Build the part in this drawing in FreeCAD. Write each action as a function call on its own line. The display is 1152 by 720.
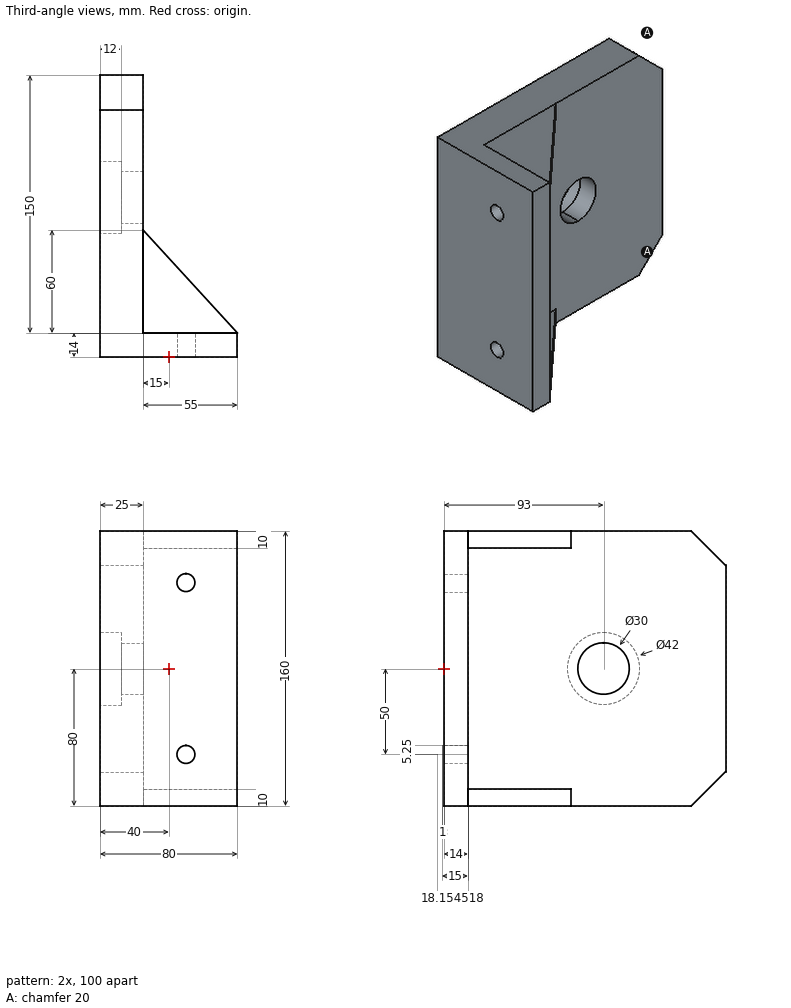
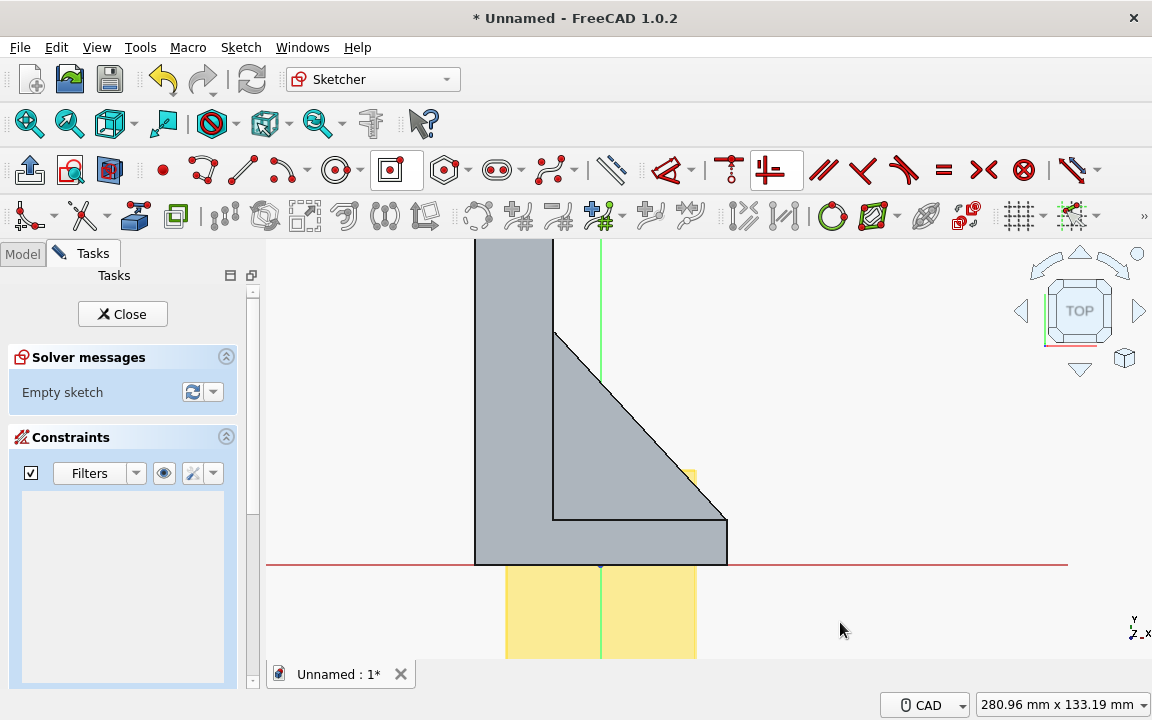
click(204, 170)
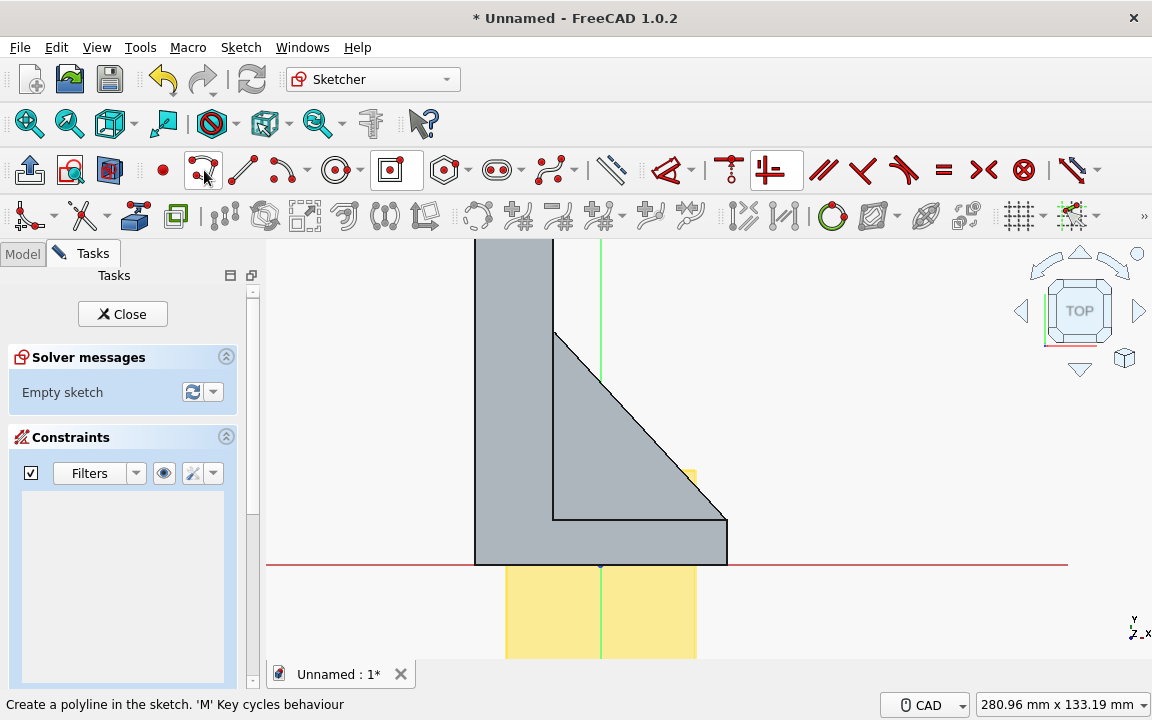
click(553, 520)
click(553, 331)
click(727, 520)
click(553, 521)
key(Escape)
key(Escape)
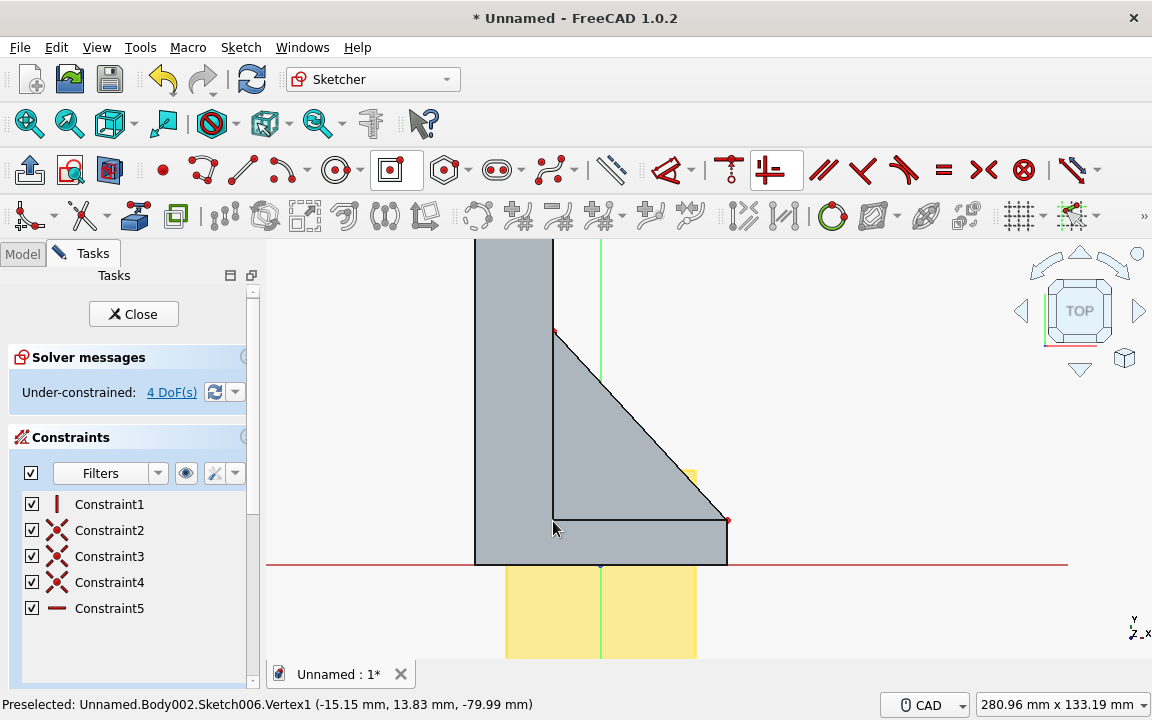
key(d)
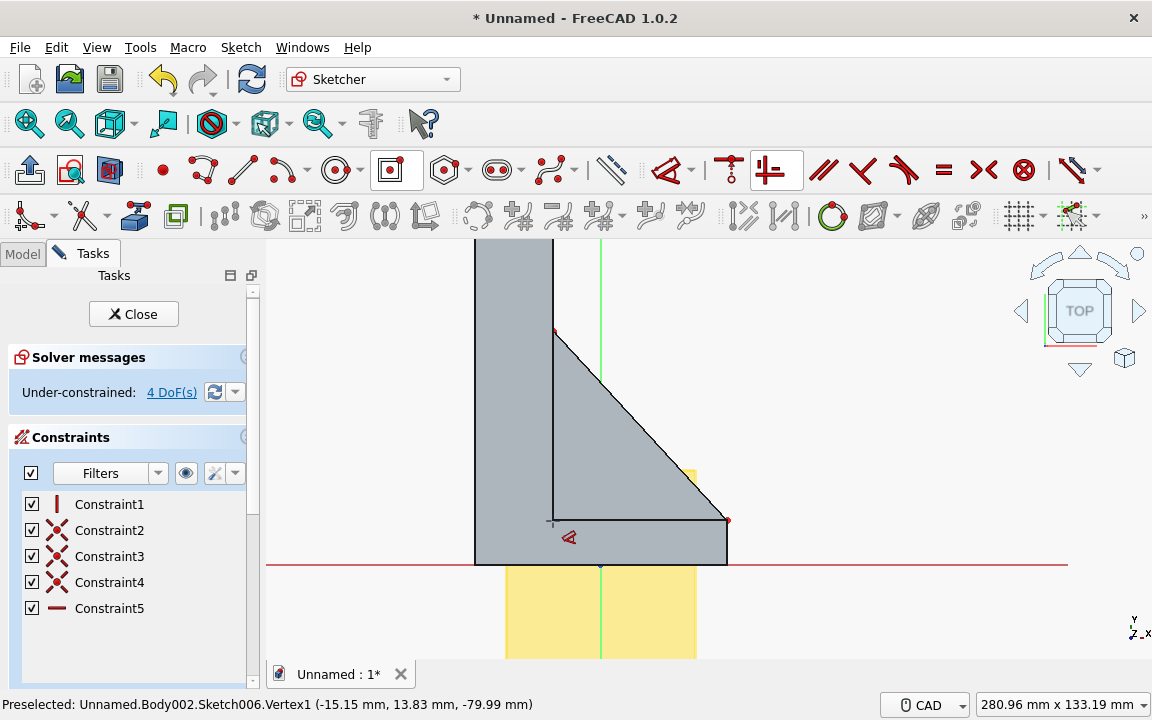
click(553, 464)
click(519, 427)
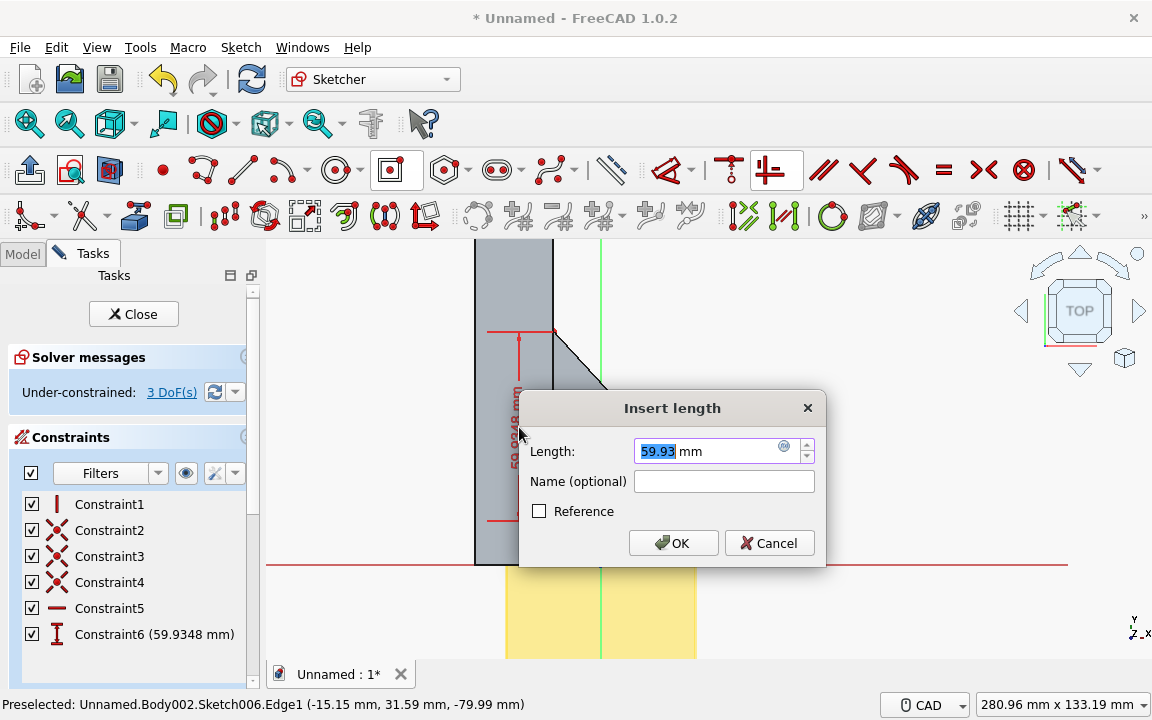
text(60)
key(Return)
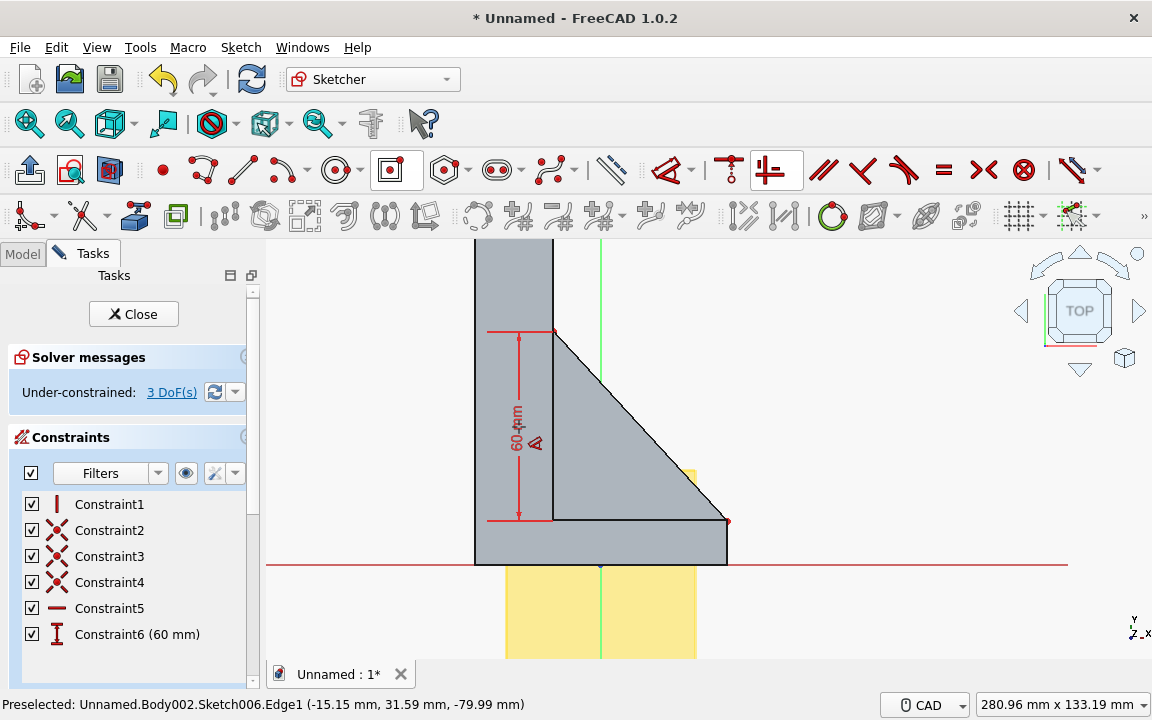
click(675, 521)
click(640, 487)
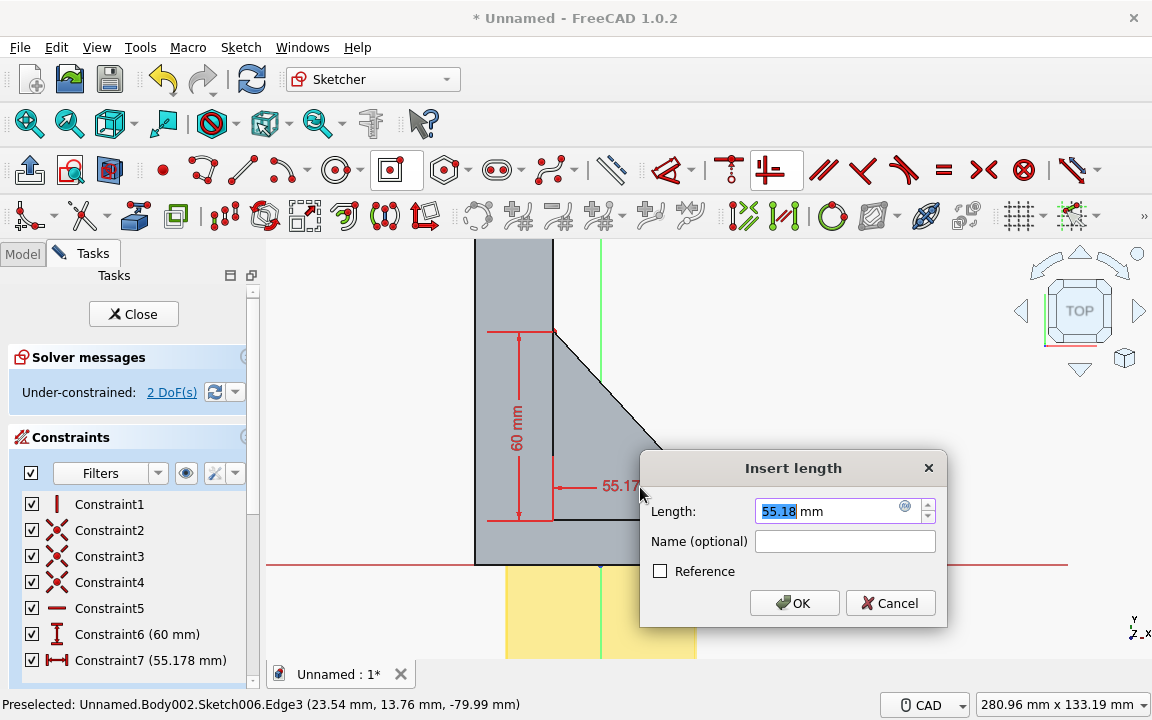
text(55)
key(Return)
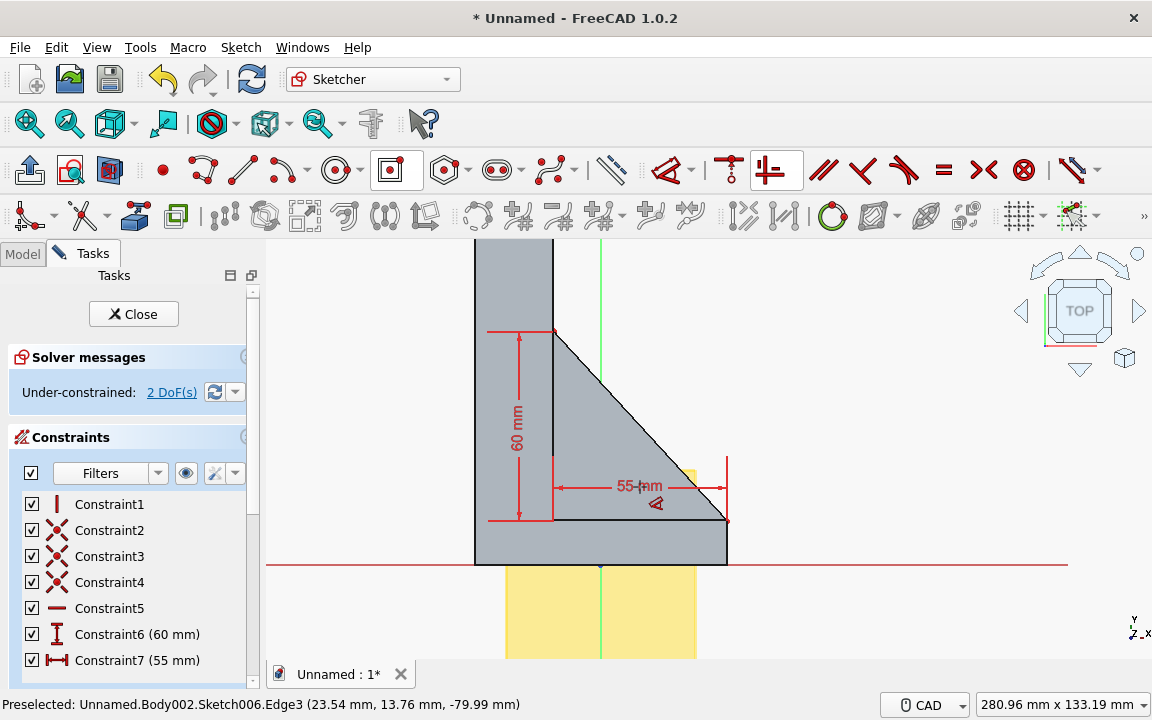
click(553, 521)
click(577, 599)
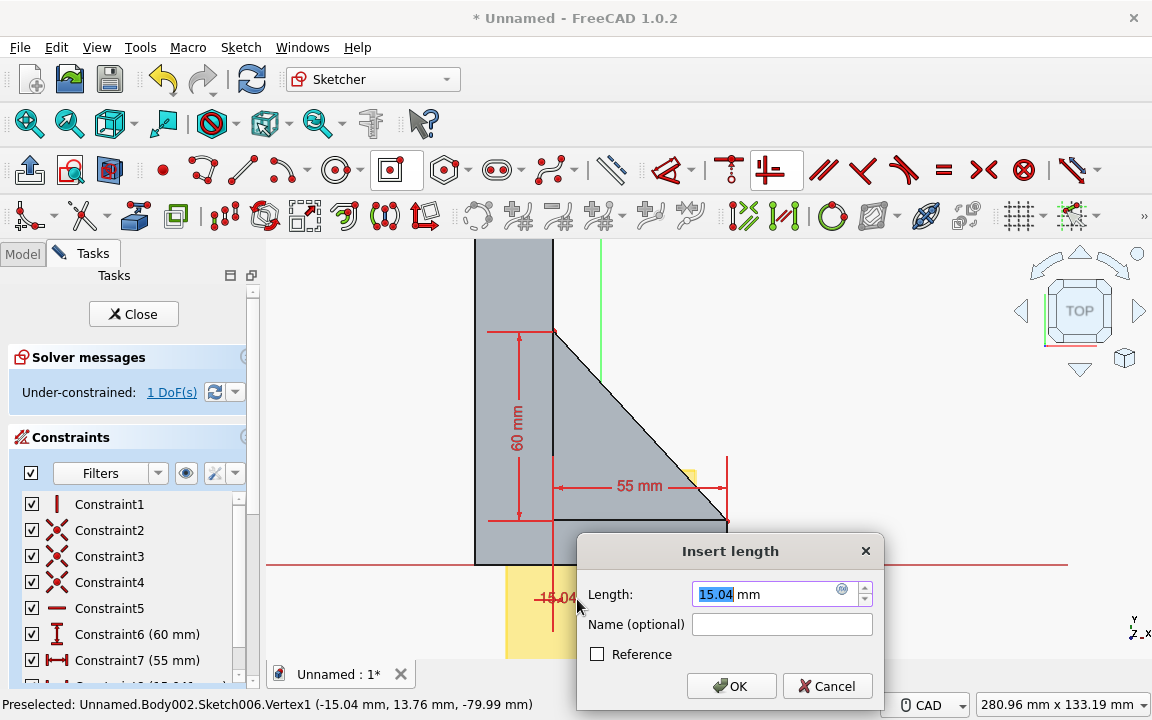
text(15)
key(Return)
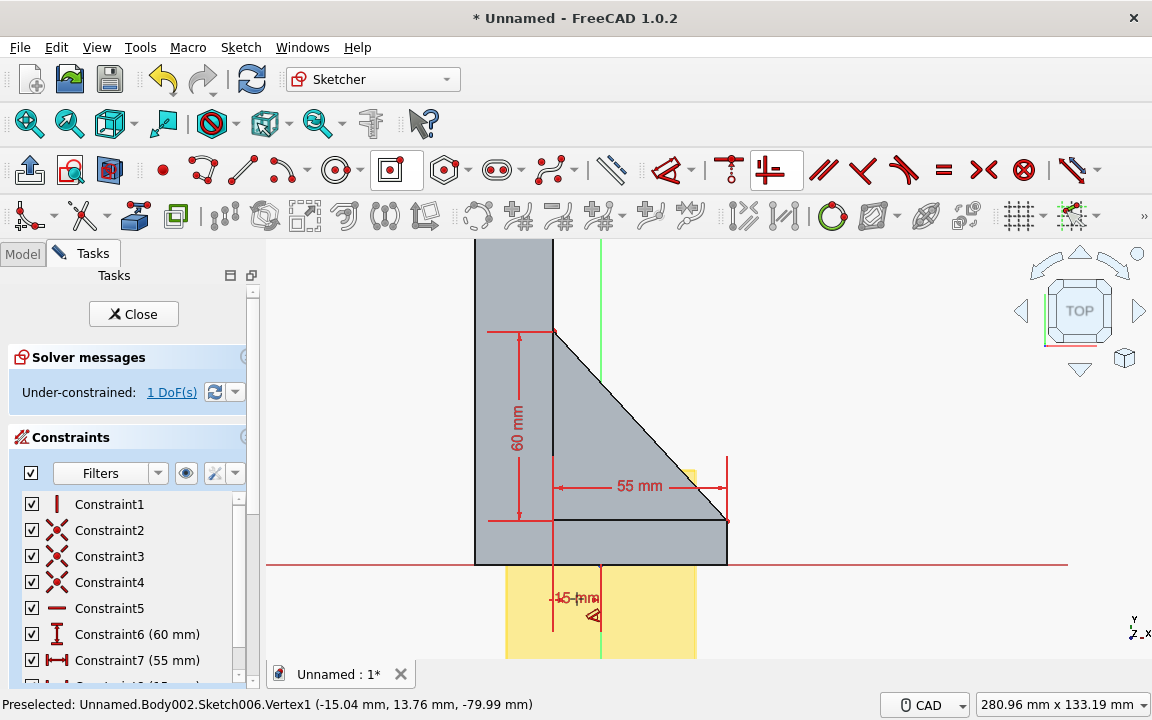
click(553, 521)
click(519, 543)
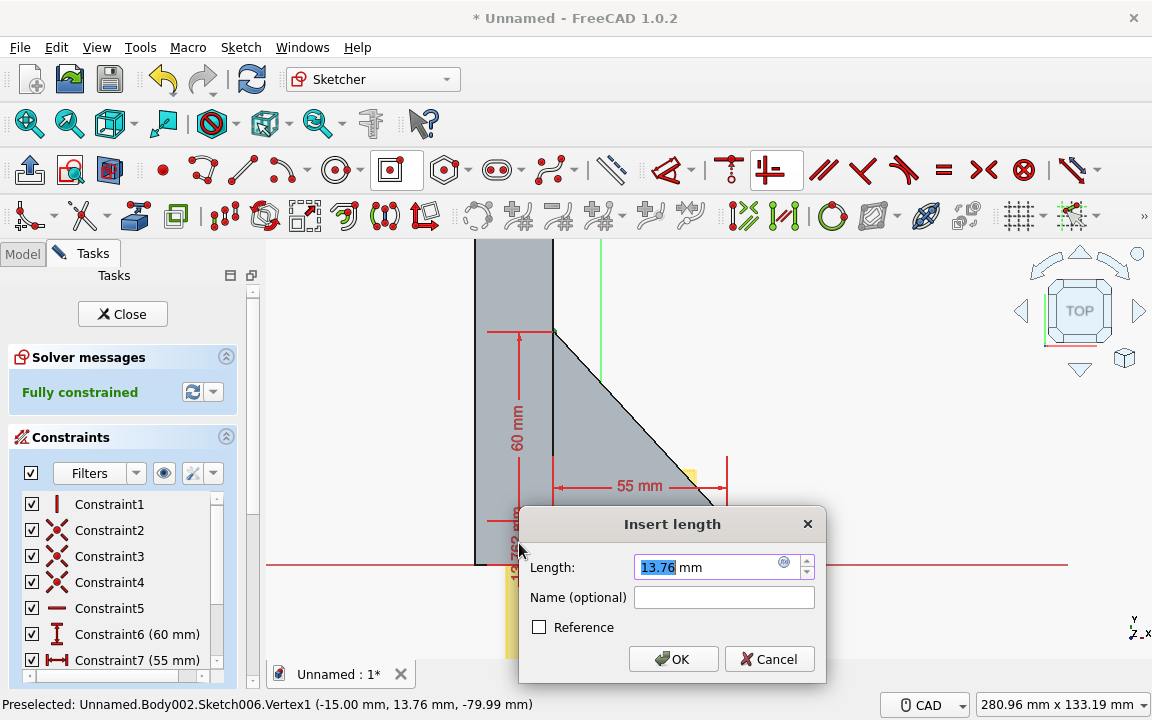
text(14)
key(Return)
key(Escape)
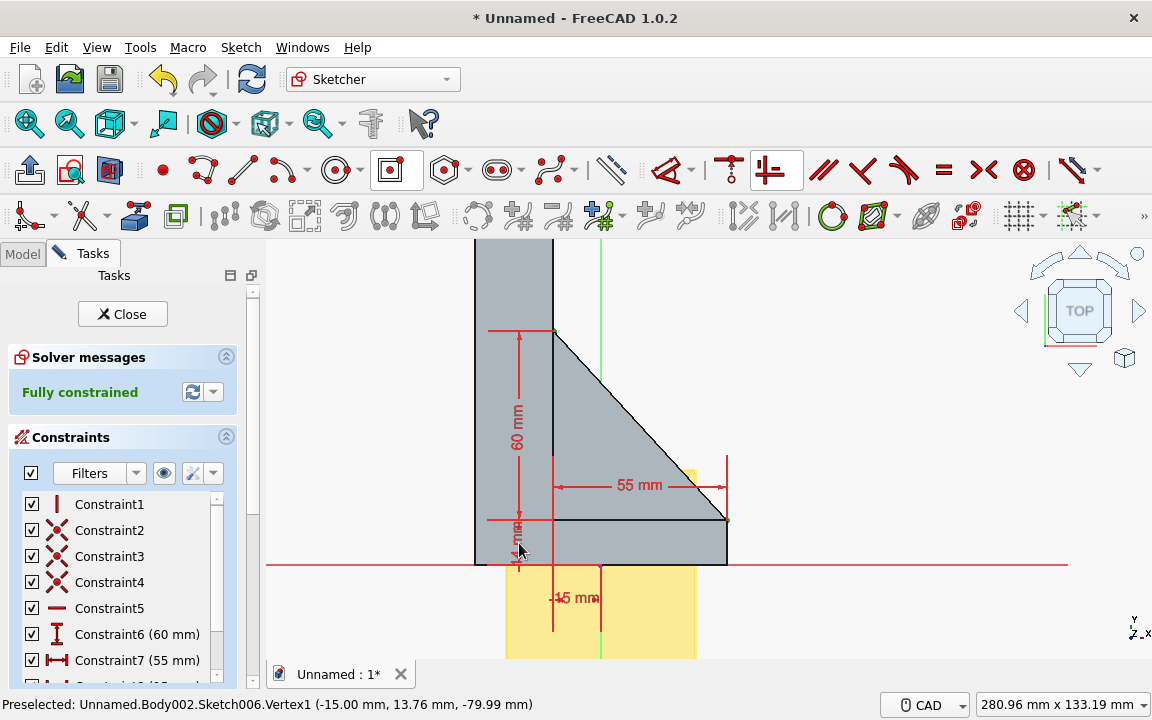
click(123, 314)